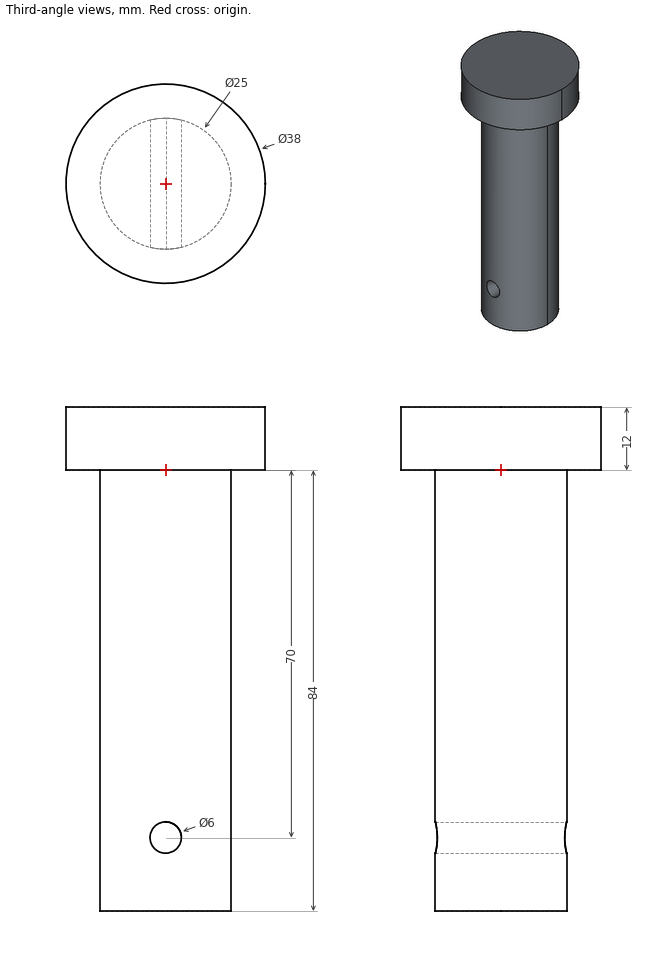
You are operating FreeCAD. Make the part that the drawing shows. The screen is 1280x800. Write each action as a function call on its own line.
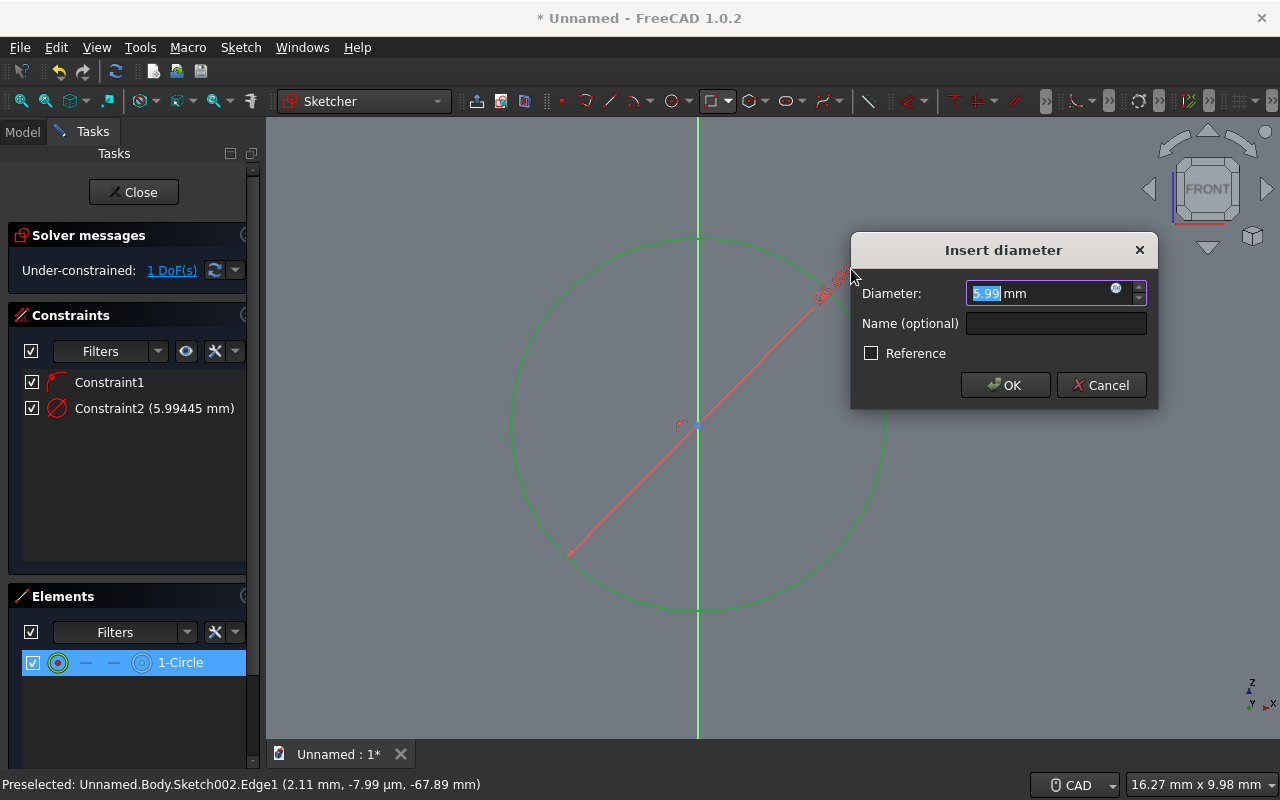
text(6)
key(Return)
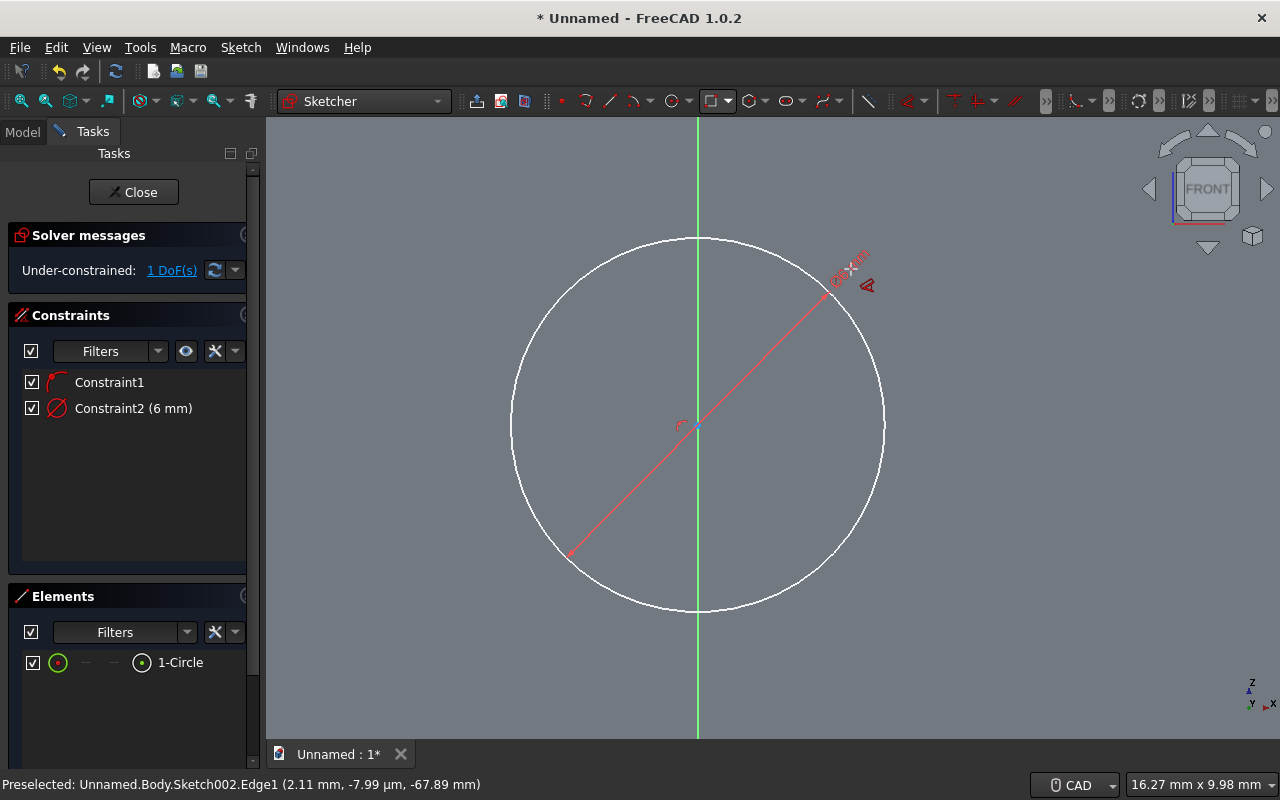
click(698, 425)
click(732, 285)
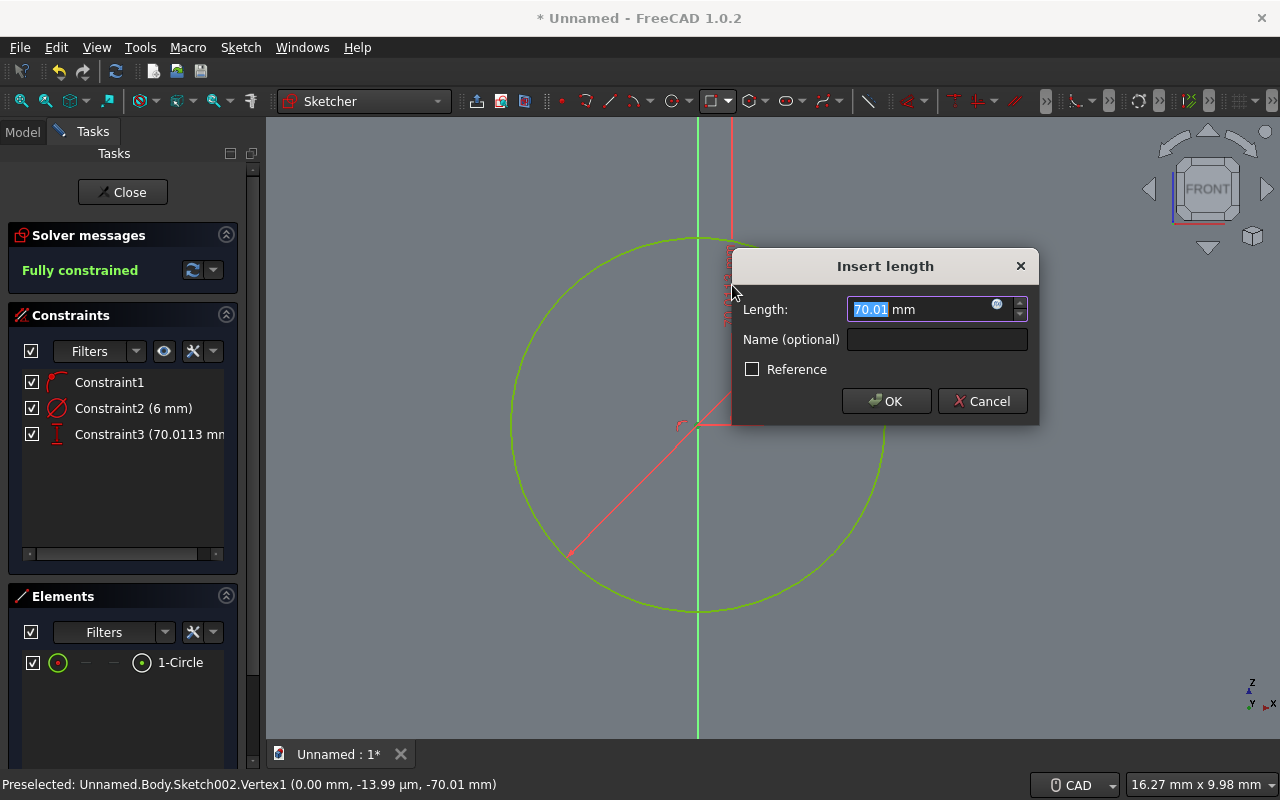
text(70)
key(Return)
key(Escape)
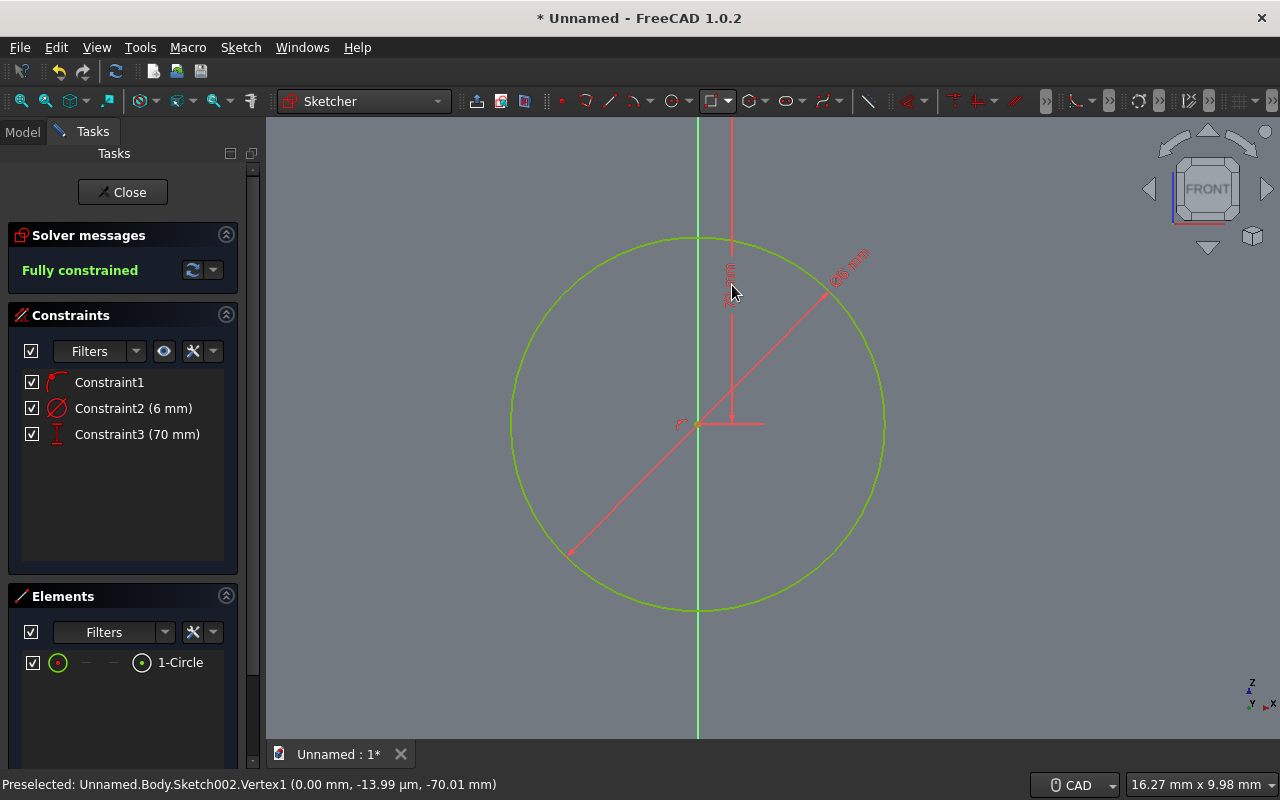
click(123, 192)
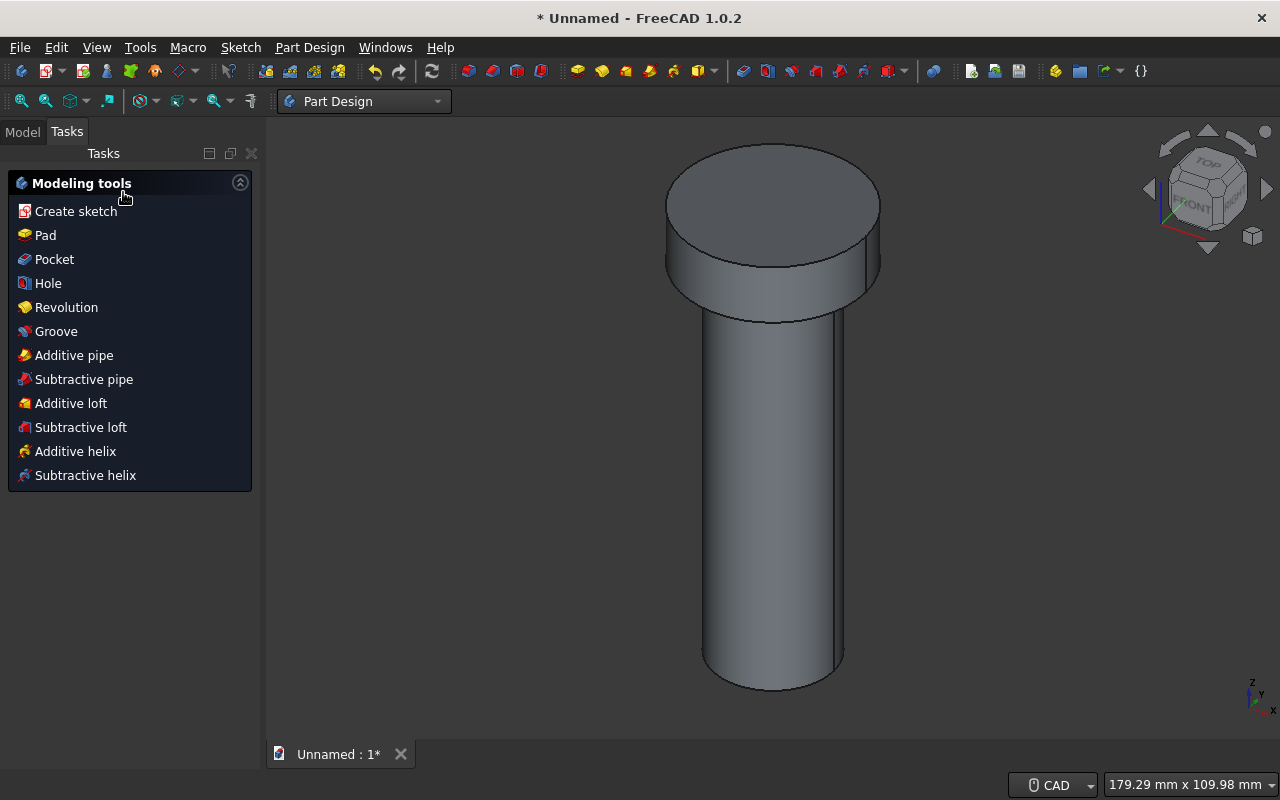
click(744, 72)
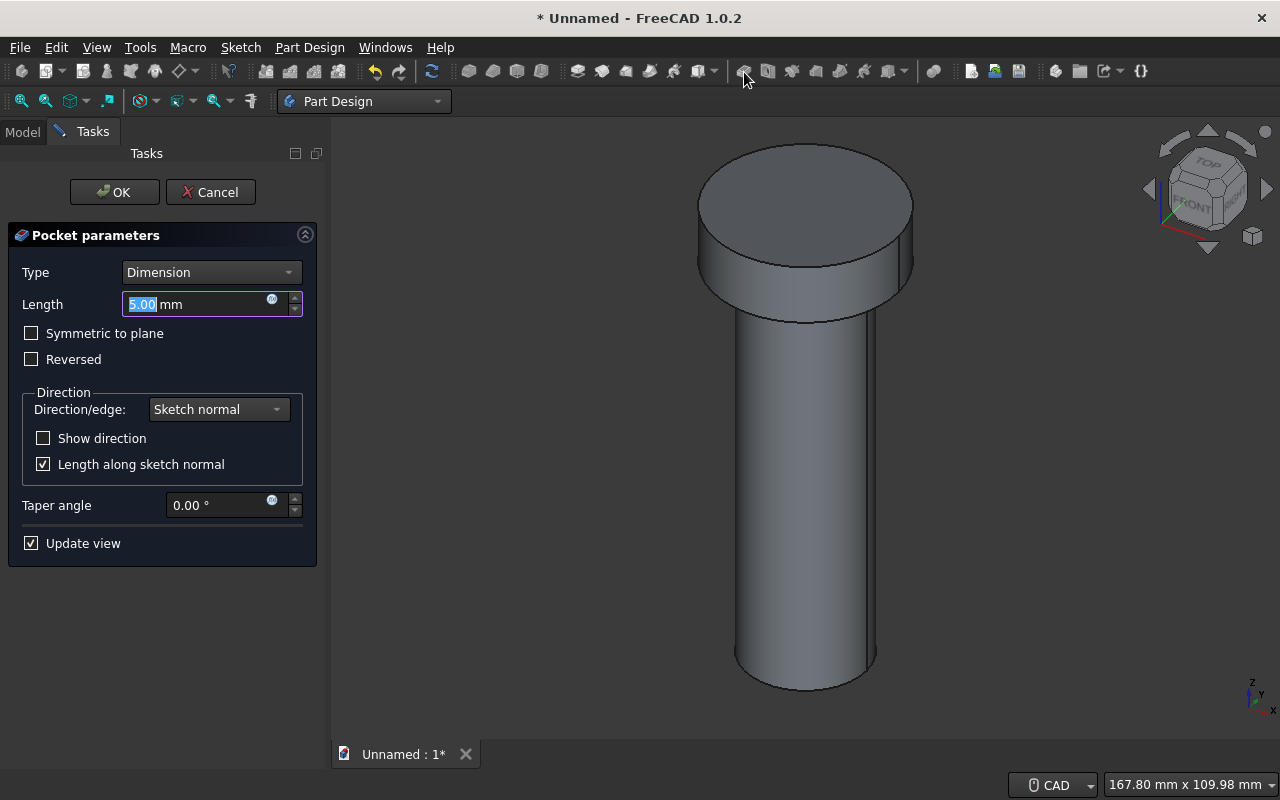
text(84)
key(Tab)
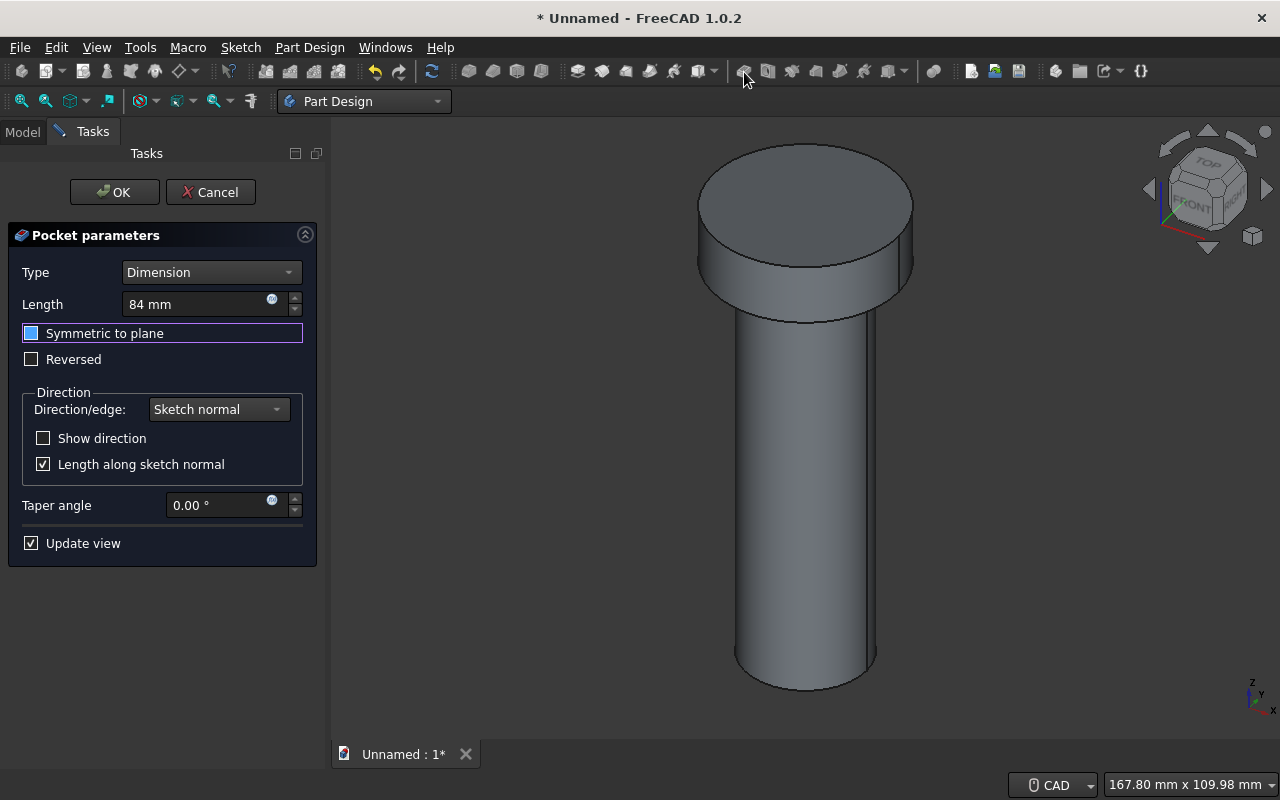
click(30, 333)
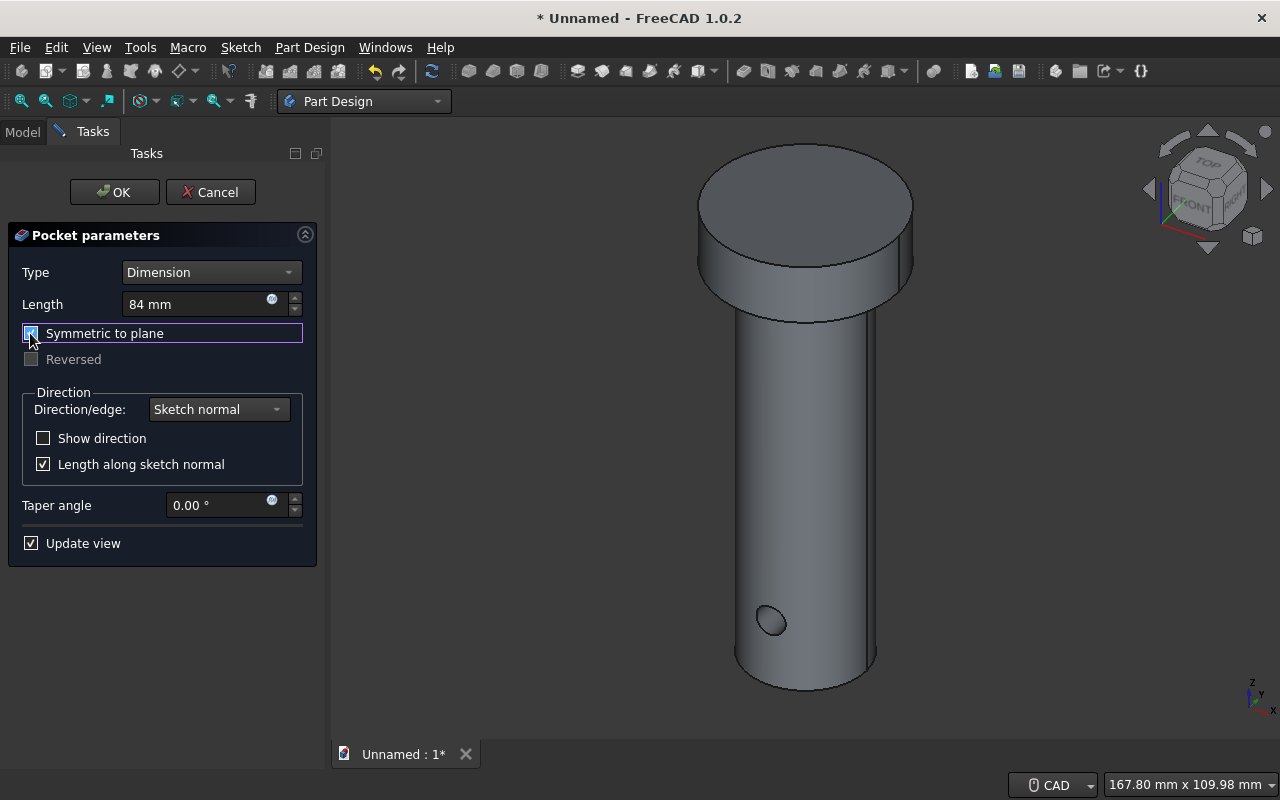
click(115, 192)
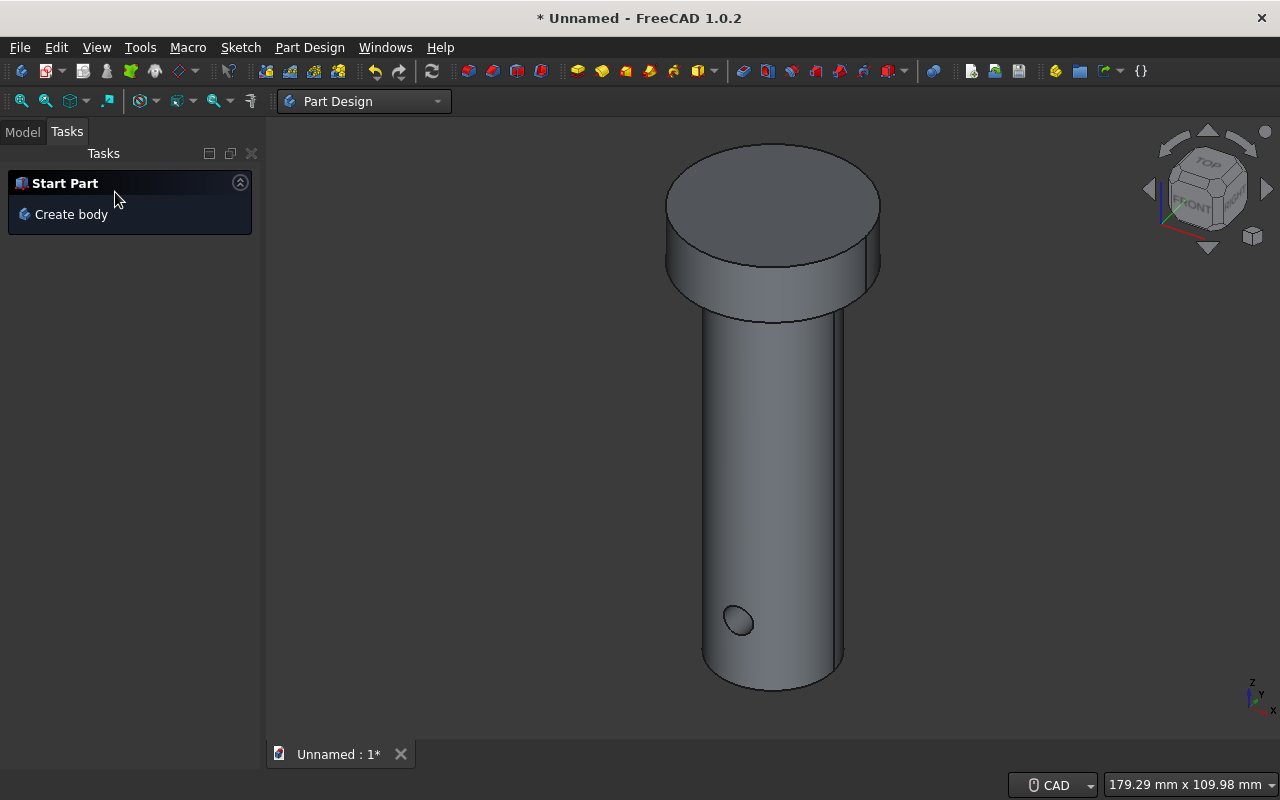
key(0)